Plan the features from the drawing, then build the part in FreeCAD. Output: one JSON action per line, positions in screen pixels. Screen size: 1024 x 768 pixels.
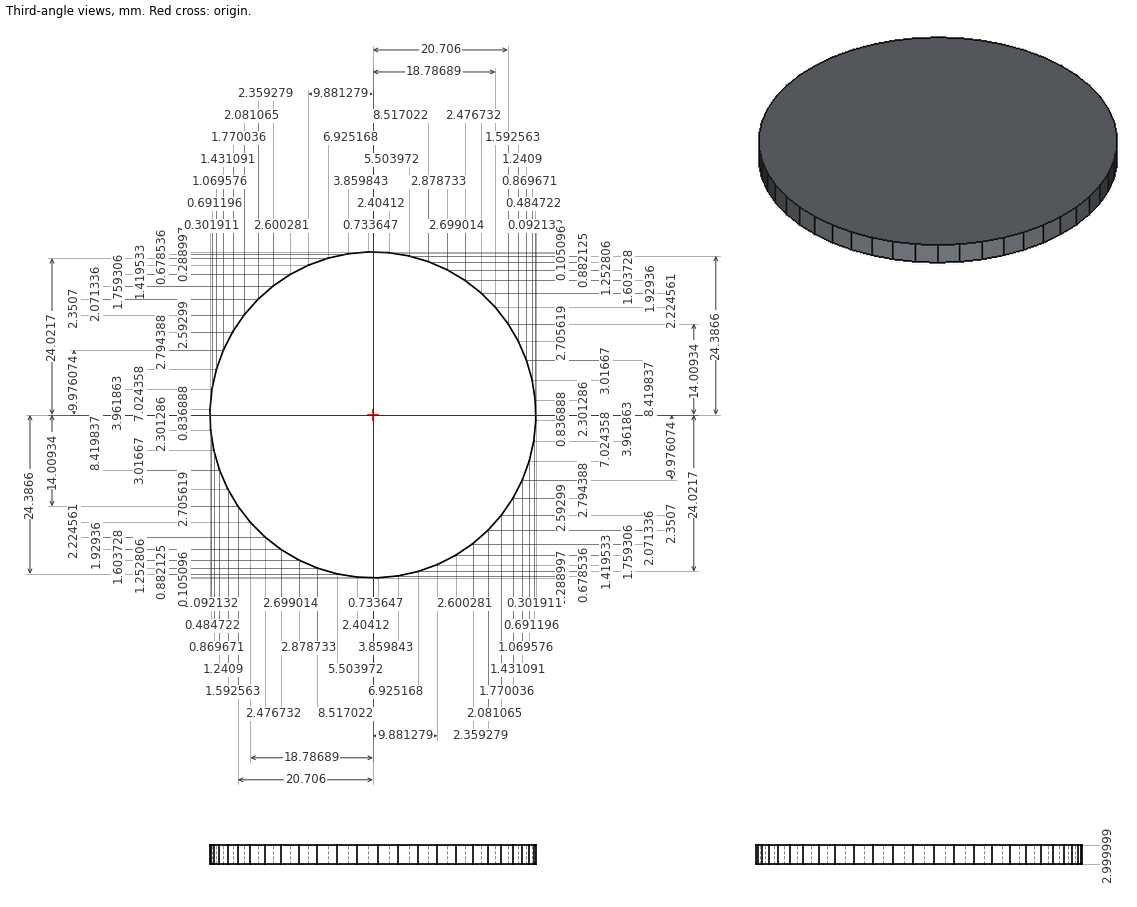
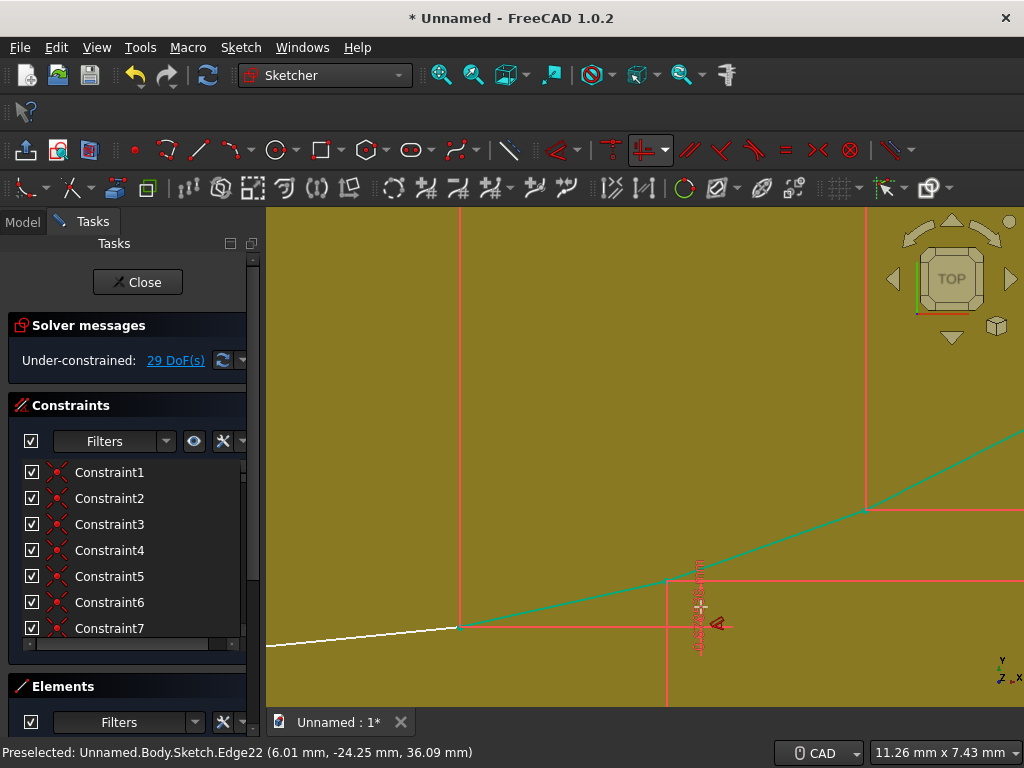
{"action": "scroll", "coordinate": [397, 633], "scroll_direction": "up", "scroll_amount": 4}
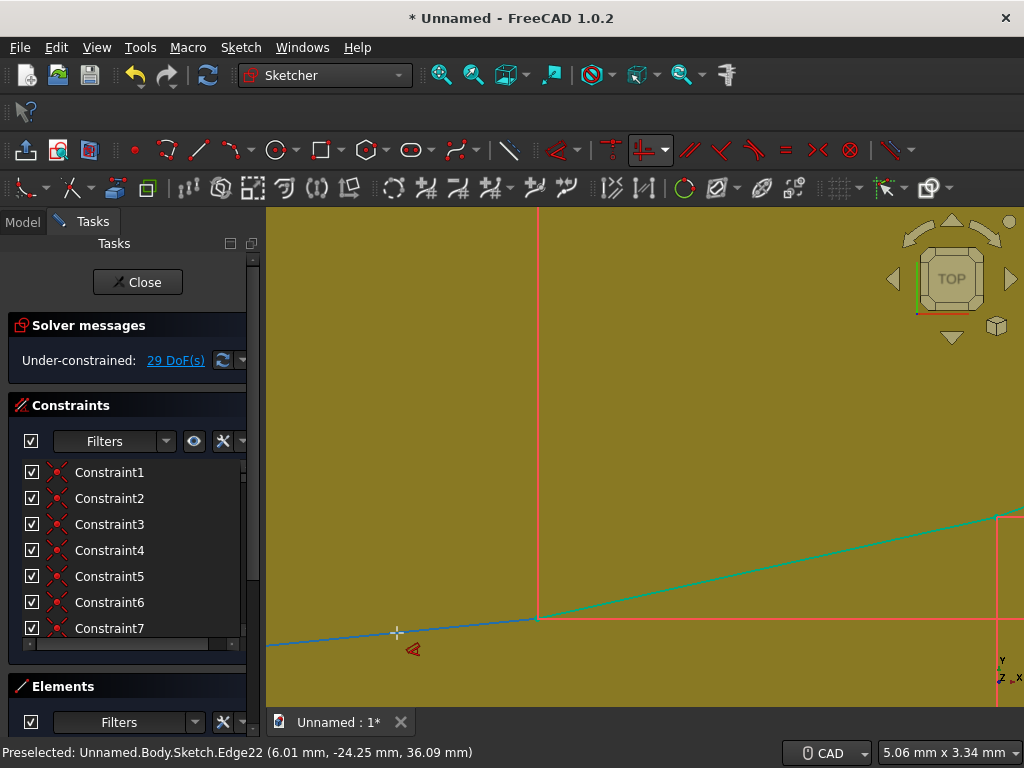
{"action": "left_click", "coordinate": [397, 633]}
{"action": "left_click", "coordinate": [572, 642]}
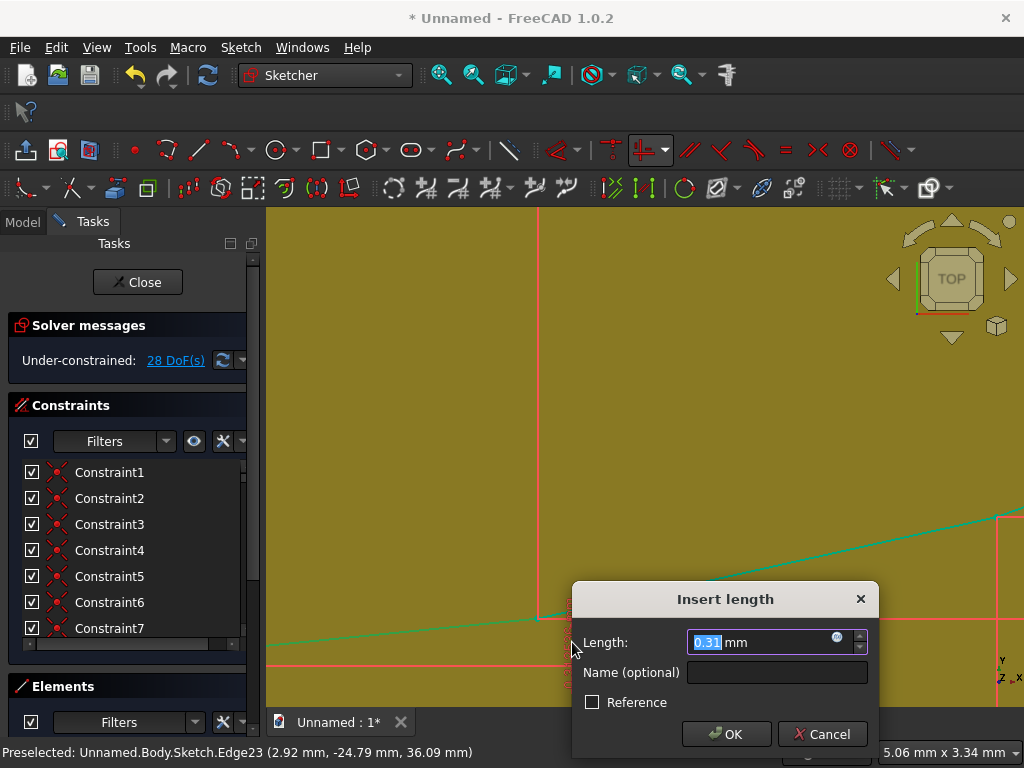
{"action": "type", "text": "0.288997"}
{"action": "key", "text": "Return"}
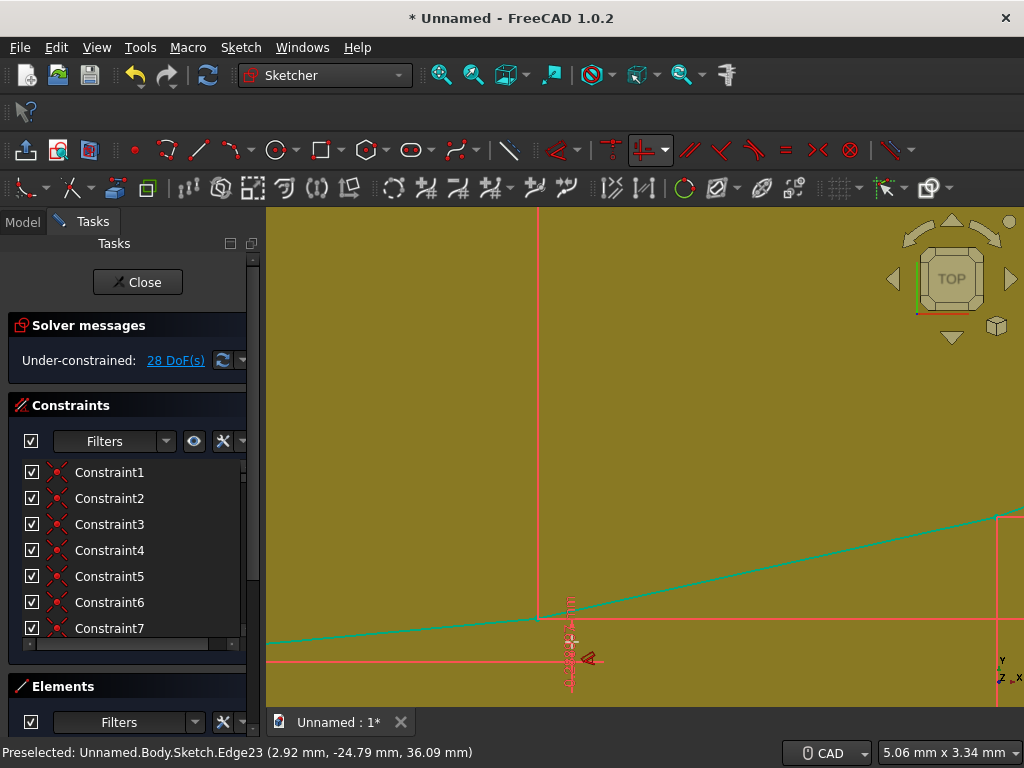
{"action": "scroll", "coordinate": [609, 642], "scroll_direction": "down", "scroll_amount": 15}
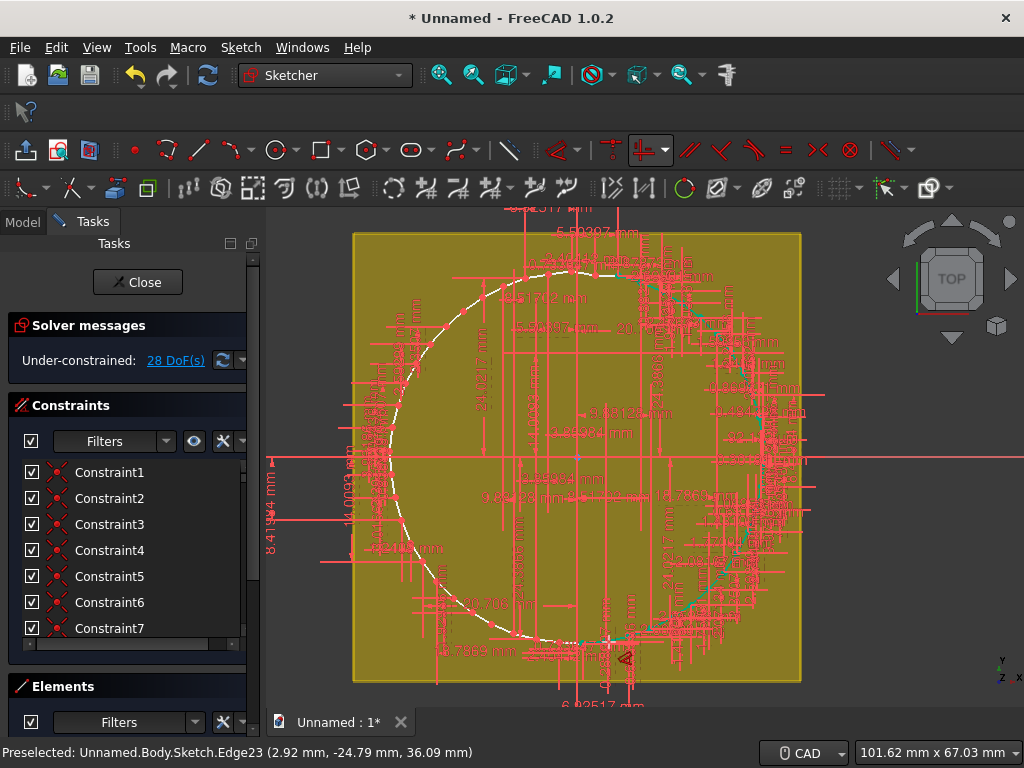
{"action": "scroll", "coordinate": [576, 643], "scroll_direction": "up", "scroll_amount": 20}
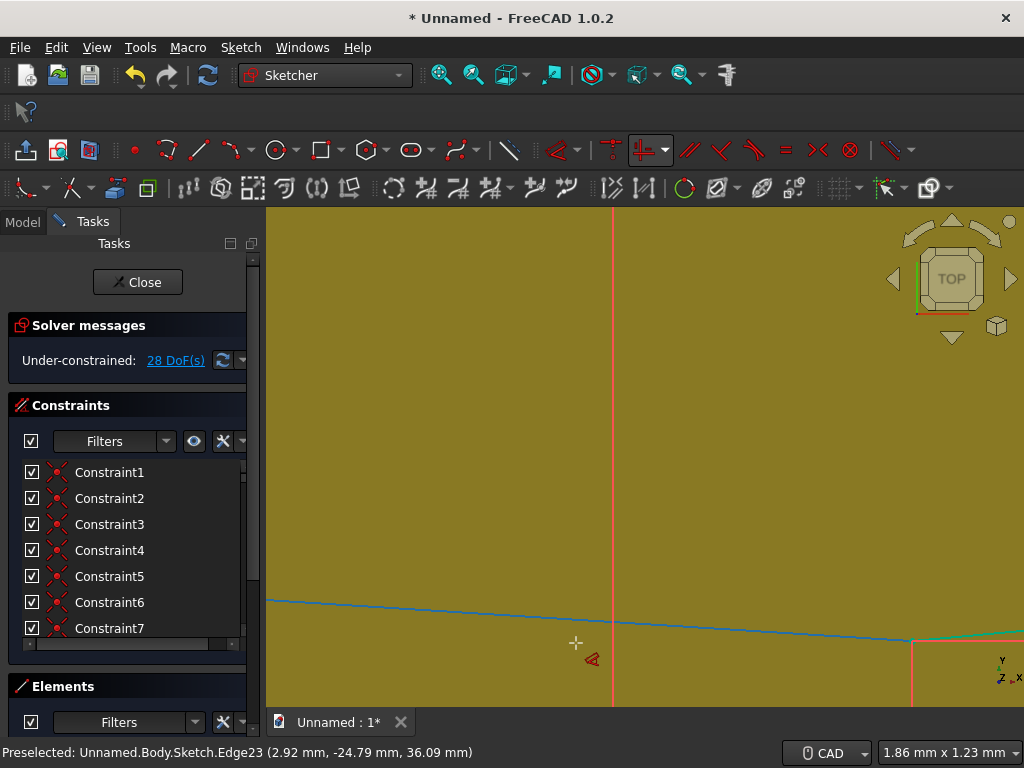
{"action": "left_click", "coordinate": [529, 617]}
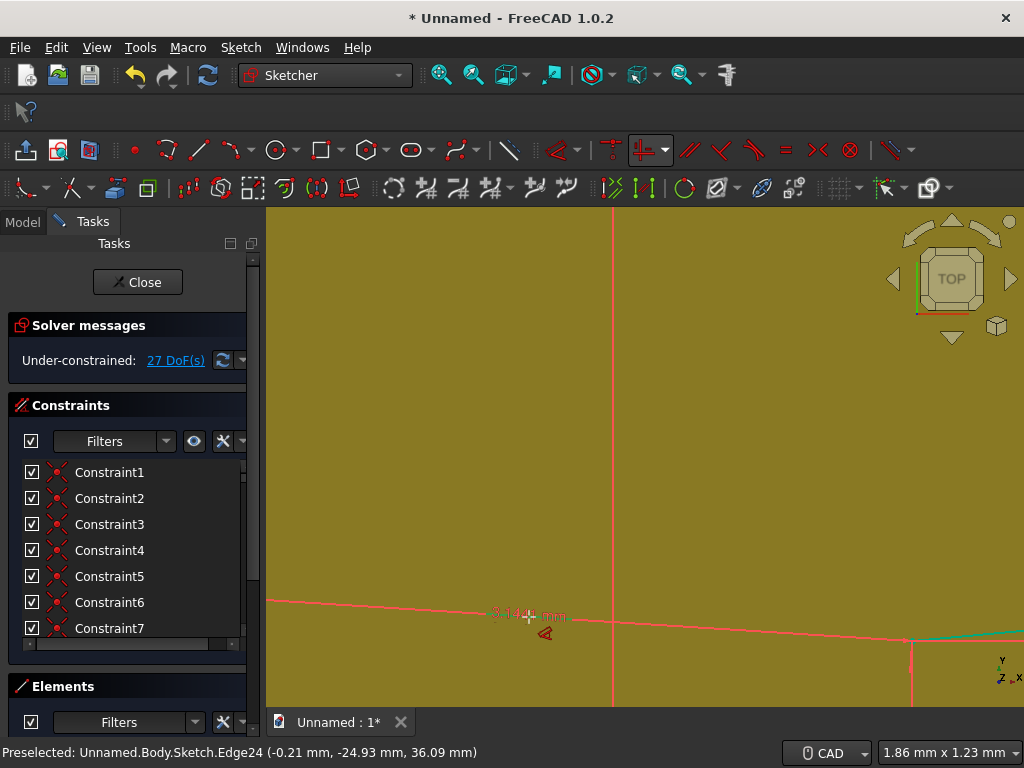
{"action": "key", "text": "Escape"}
{"action": "key", "text": "Escape"}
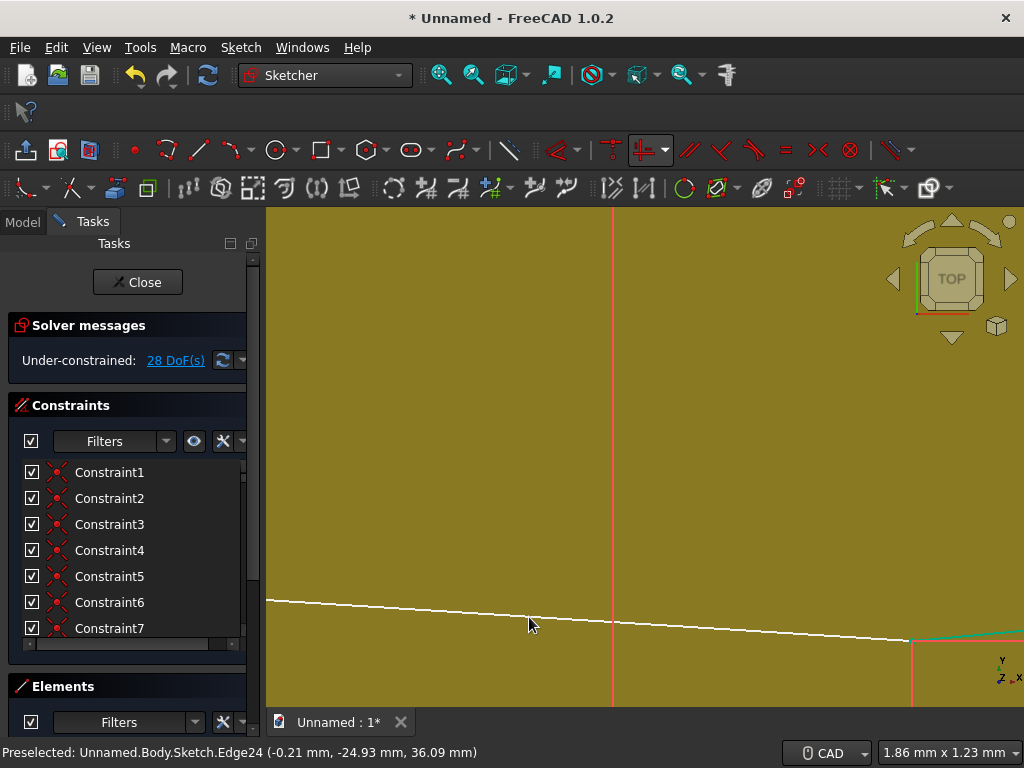
{"action": "left_click", "coordinate": [529, 617]}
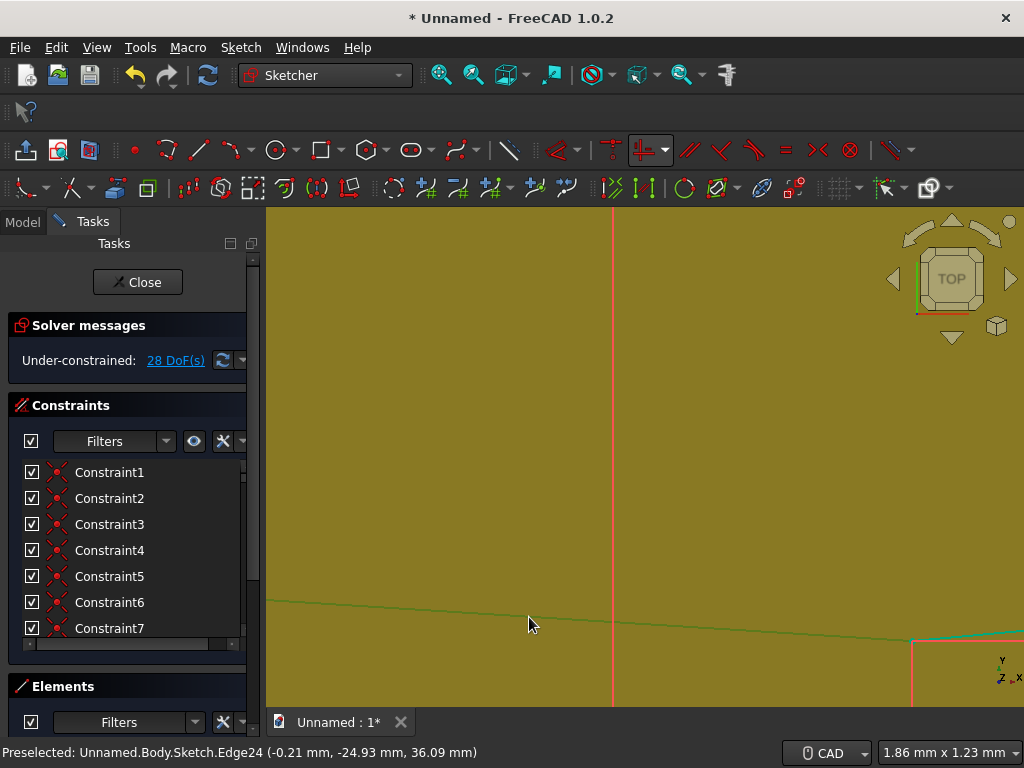
{"action": "left_click", "coordinate": [580, 150]}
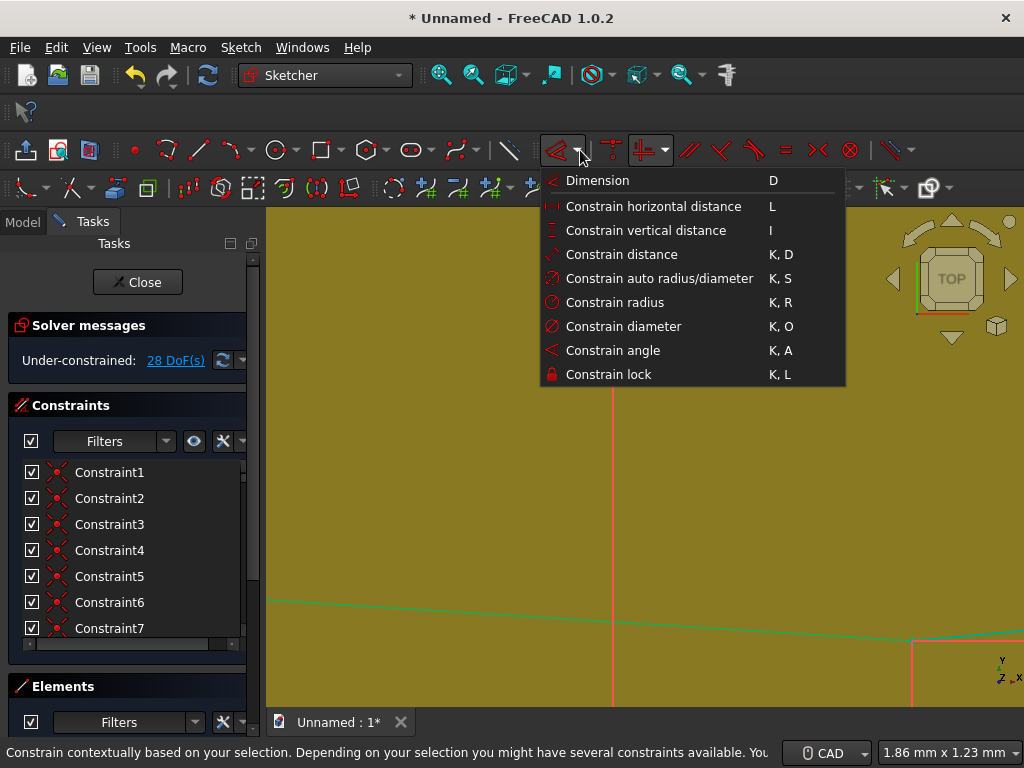
{"action": "left_click", "coordinate": [693, 230]}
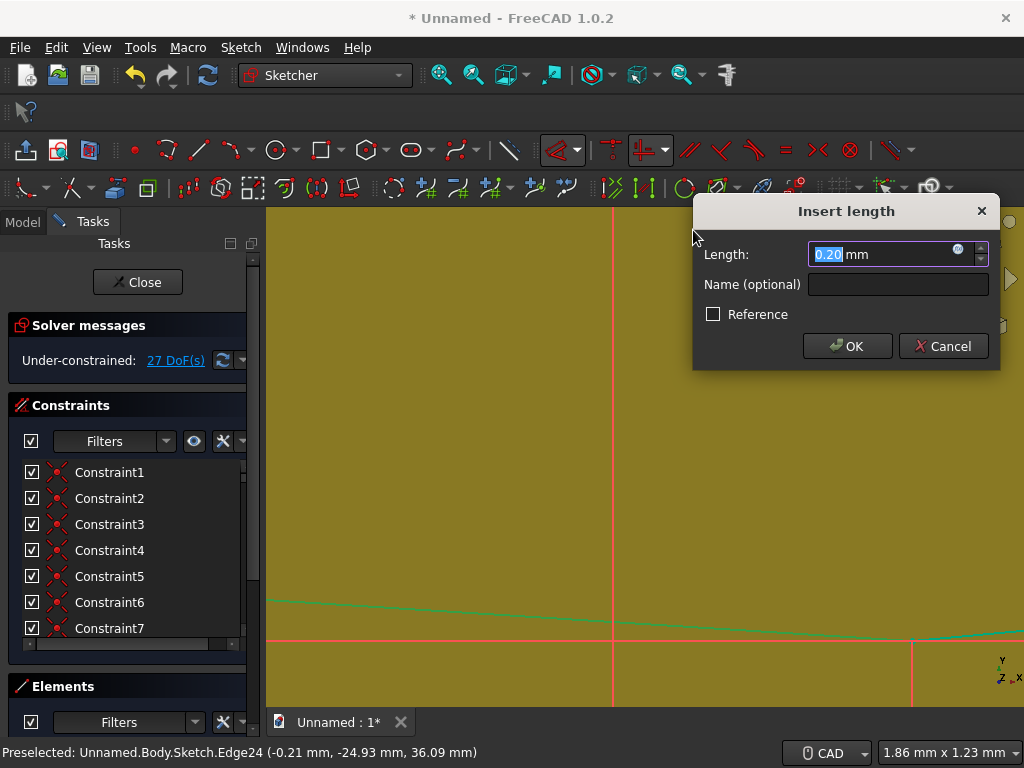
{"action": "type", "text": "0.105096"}
{"action": "key", "text": "Return"}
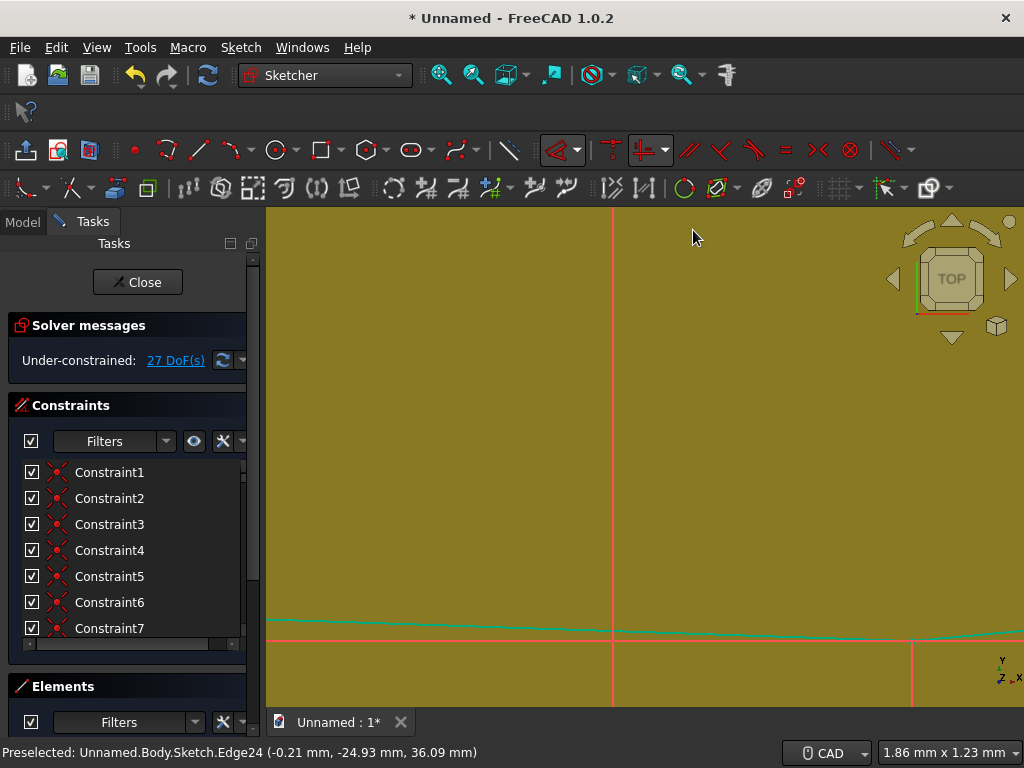
{"action": "scroll", "coordinate": [576, 457], "scroll_direction": "down", "scroll_amount": 15}